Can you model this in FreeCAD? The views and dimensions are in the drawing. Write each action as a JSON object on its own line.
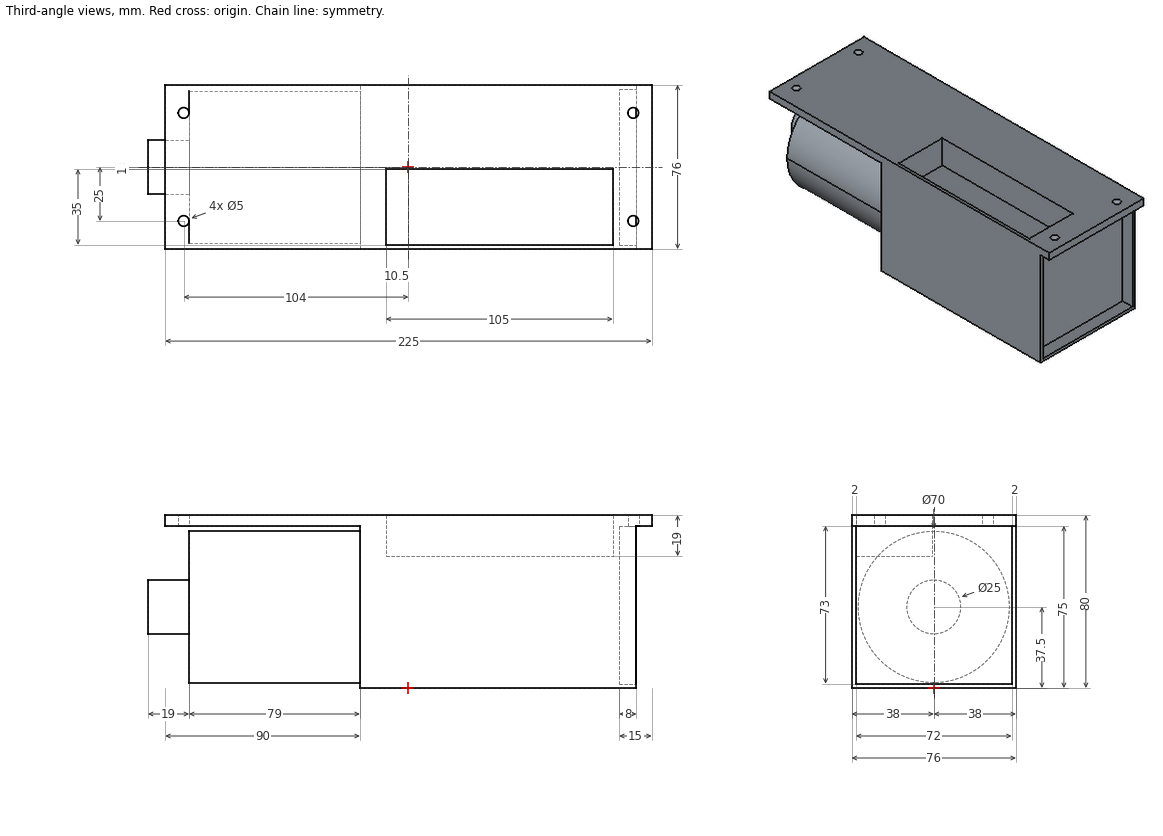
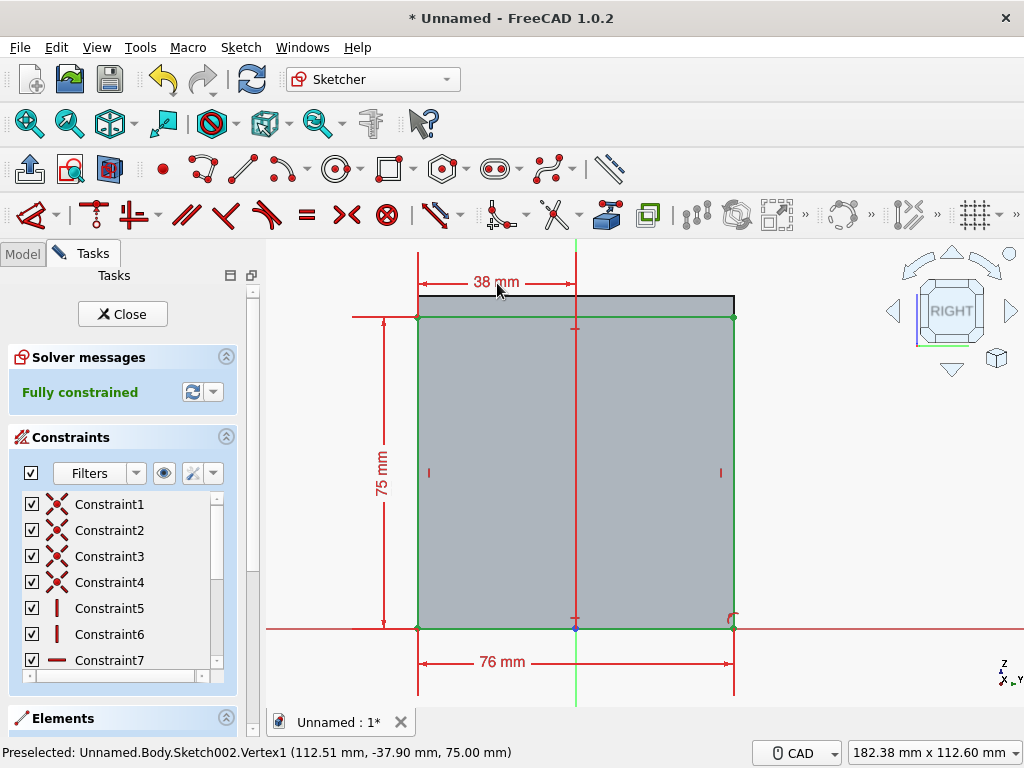
{"action": "left_click", "coordinate": [123, 314]}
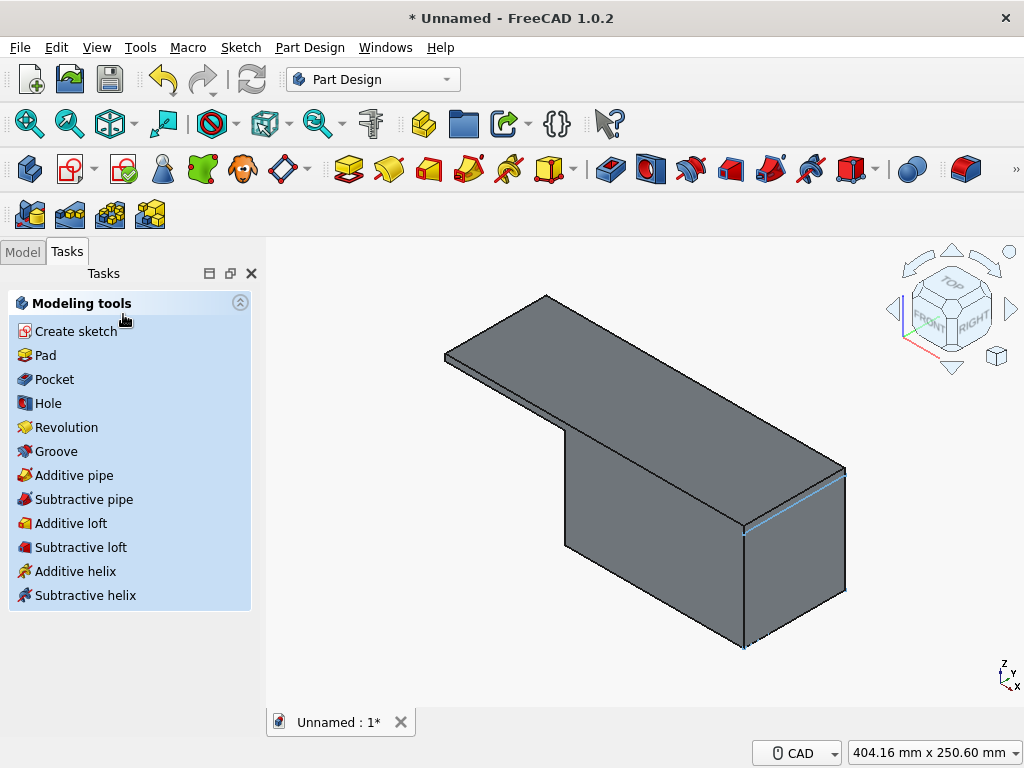
{"action": "left_click", "coordinate": [612, 170]}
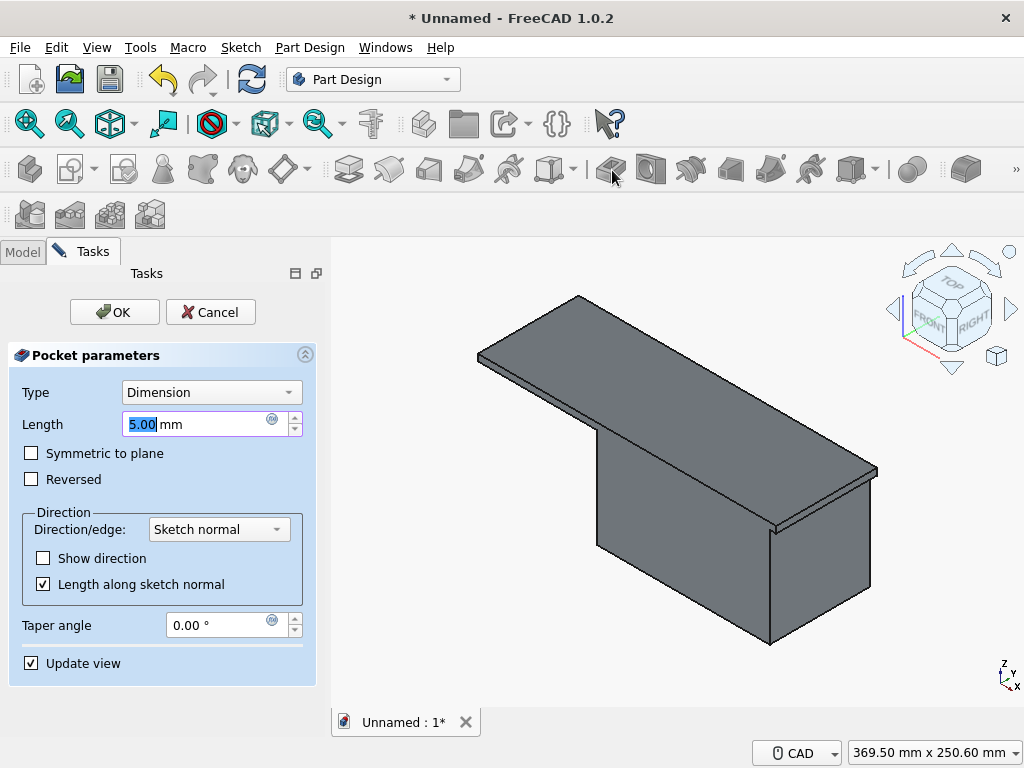
{"action": "type", "text": "15"}
{"action": "key", "text": "Tab"}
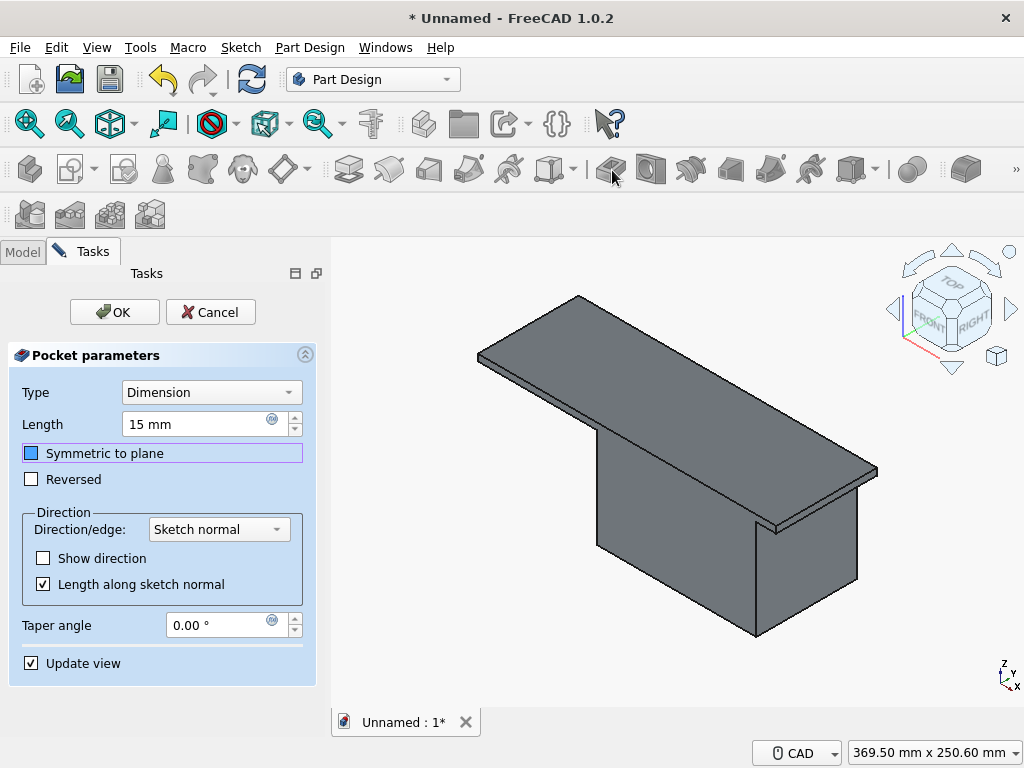
{"action": "left_click", "coordinate": [115, 312]}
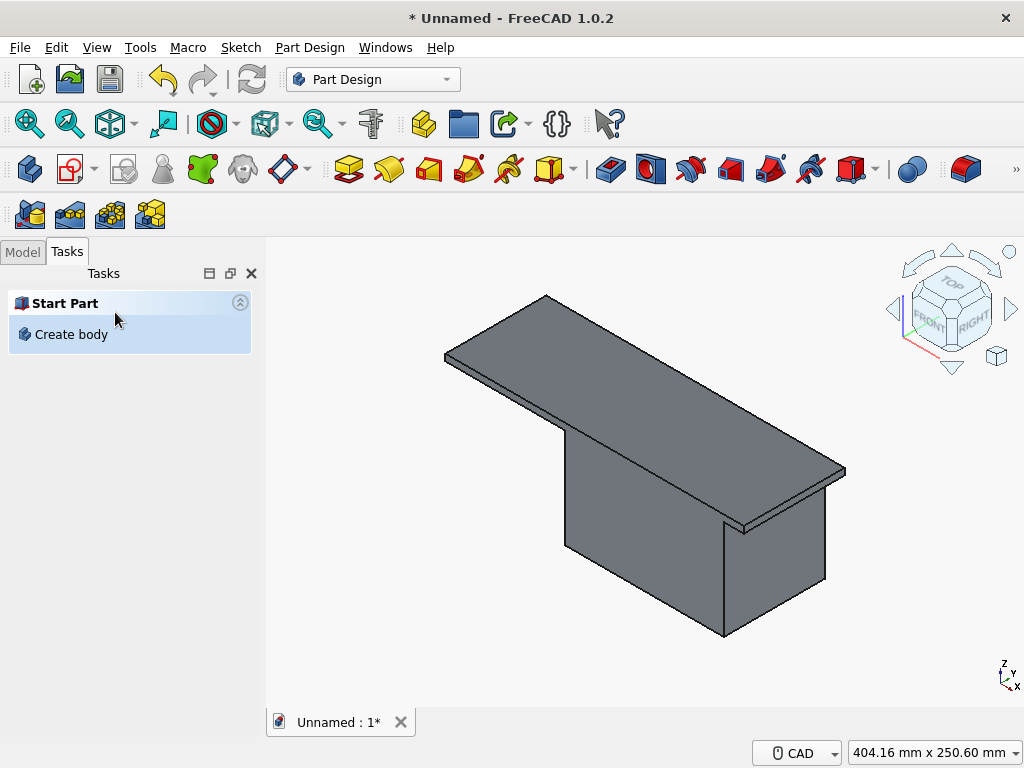
{"action": "key", "text": "5"}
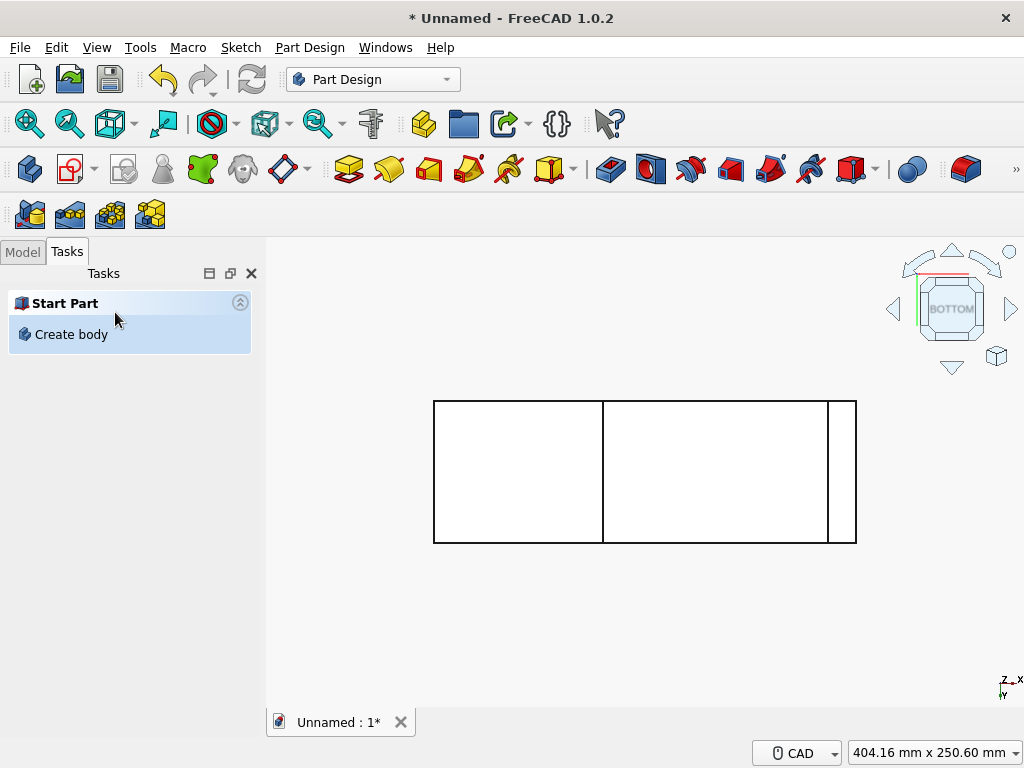
{"action": "left_click", "coordinate": [518, 471]}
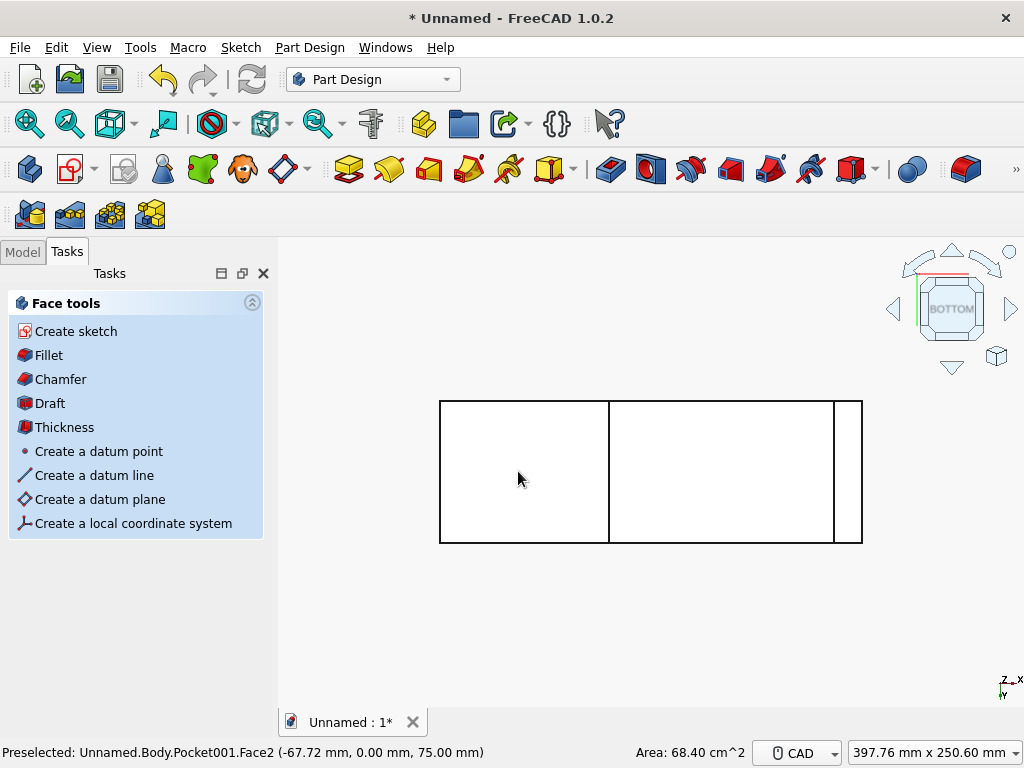
{"action": "left_click", "coordinate": [70, 170]}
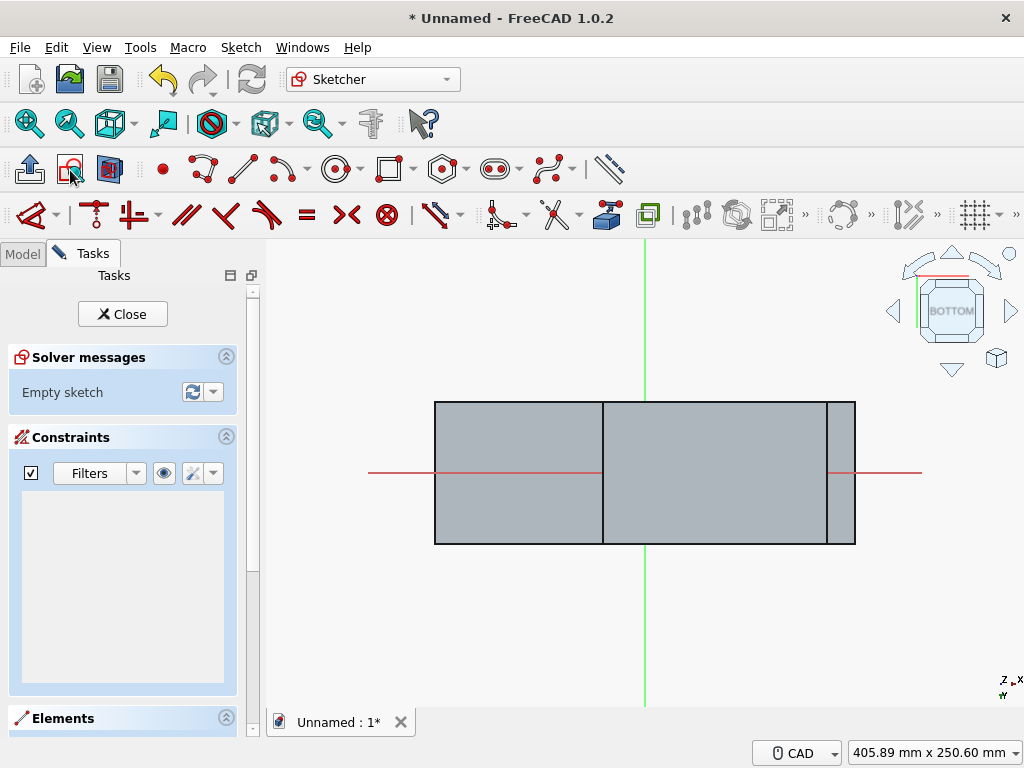
{"action": "scroll", "coordinate": [294, 473], "scroll_direction": "down", "scroll_amount": 1}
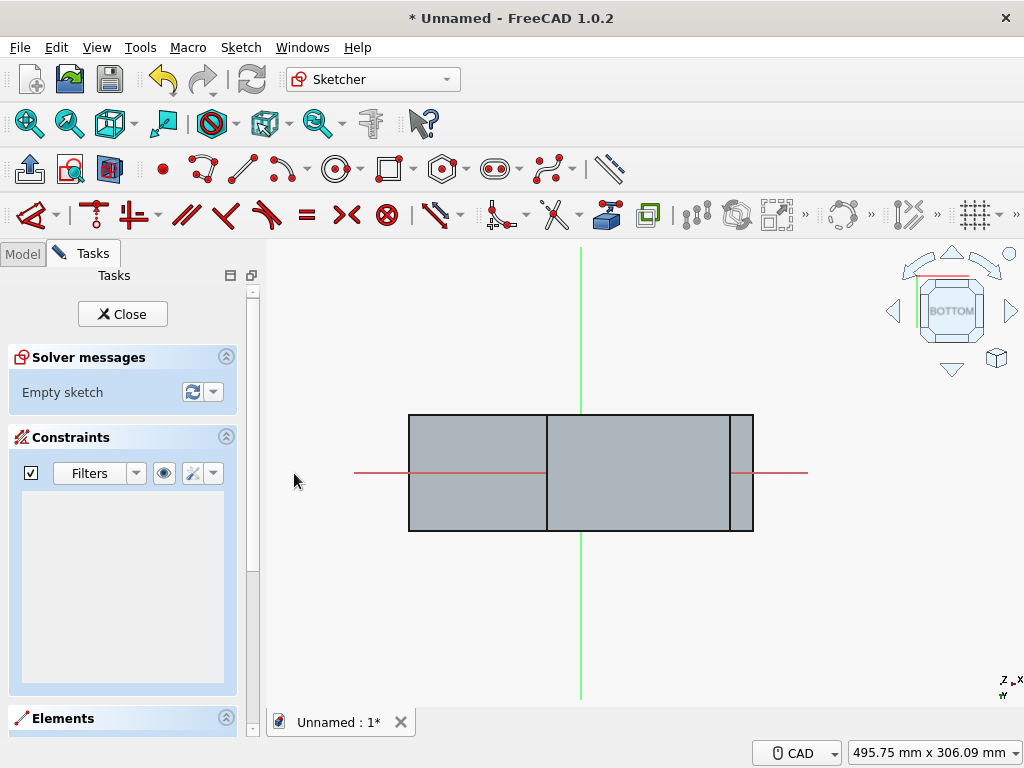
{"action": "key", "text": "g c"}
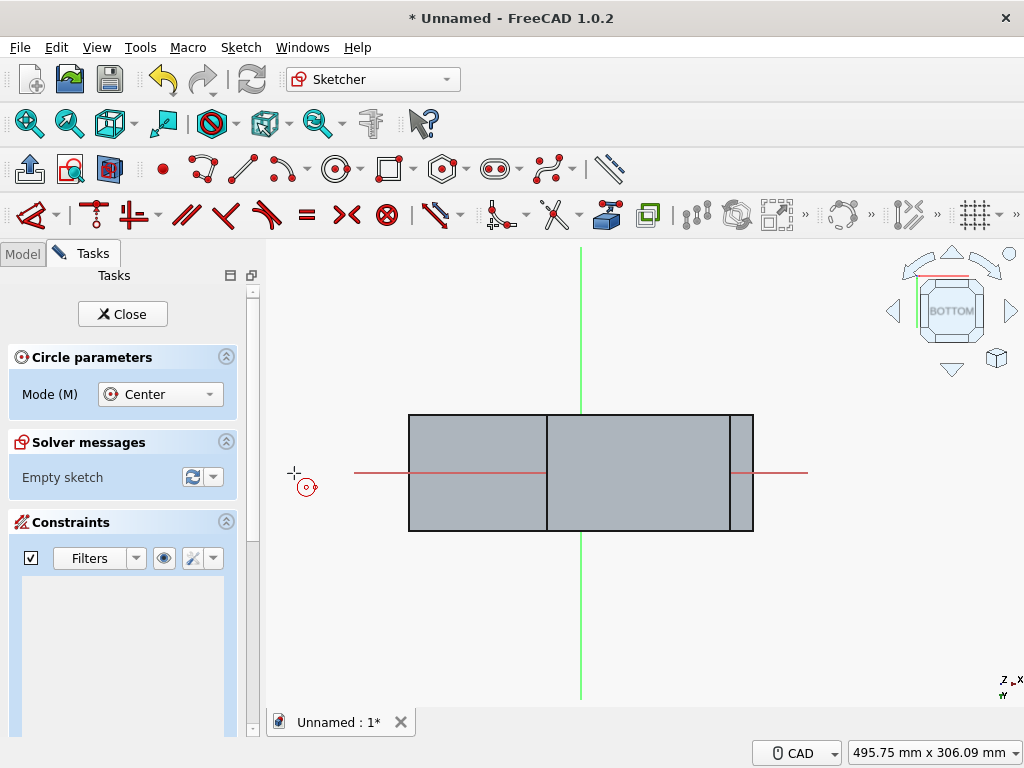
{"action": "scroll", "coordinate": [422, 435], "scroll_direction": "up", "scroll_amount": 9}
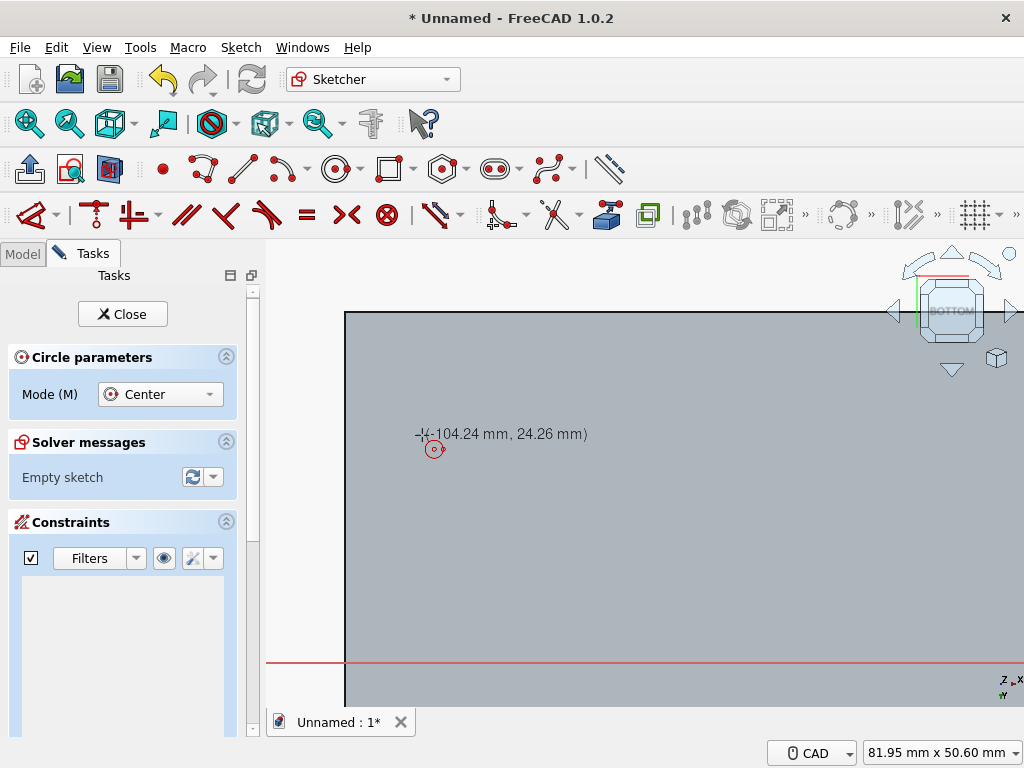
{"action": "scroll", "coordinate": [372, 425], "scroll_direction": "down", "scroll_amount": 8}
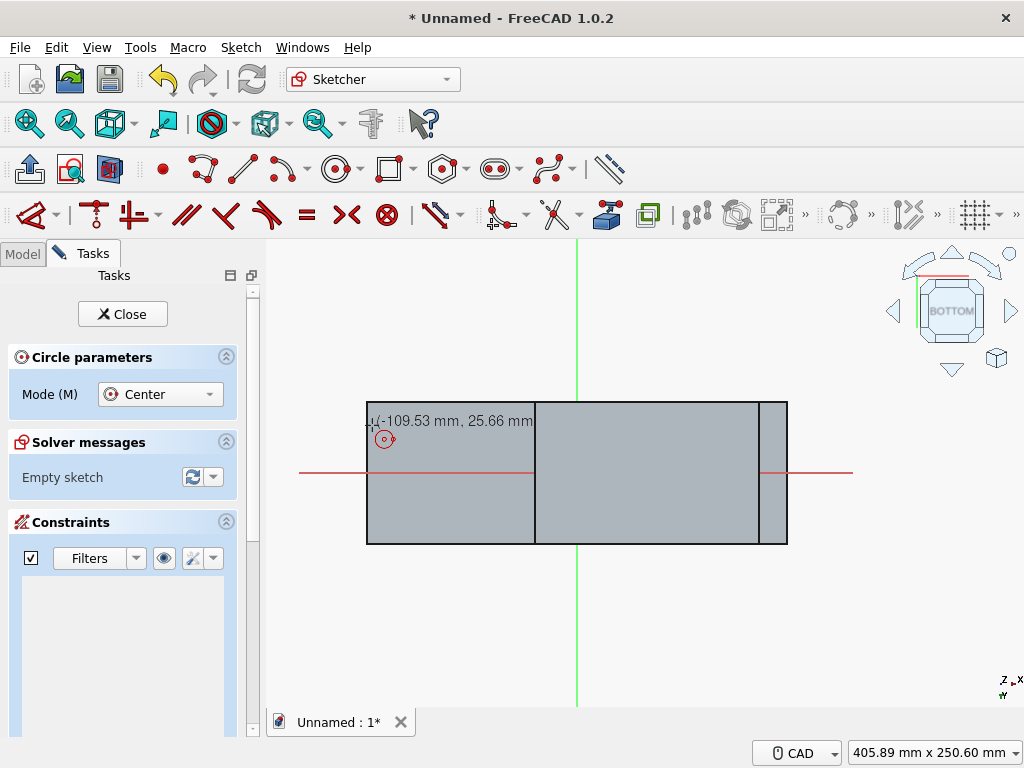
{"action": "left_click", "coordinate": [382, 427]}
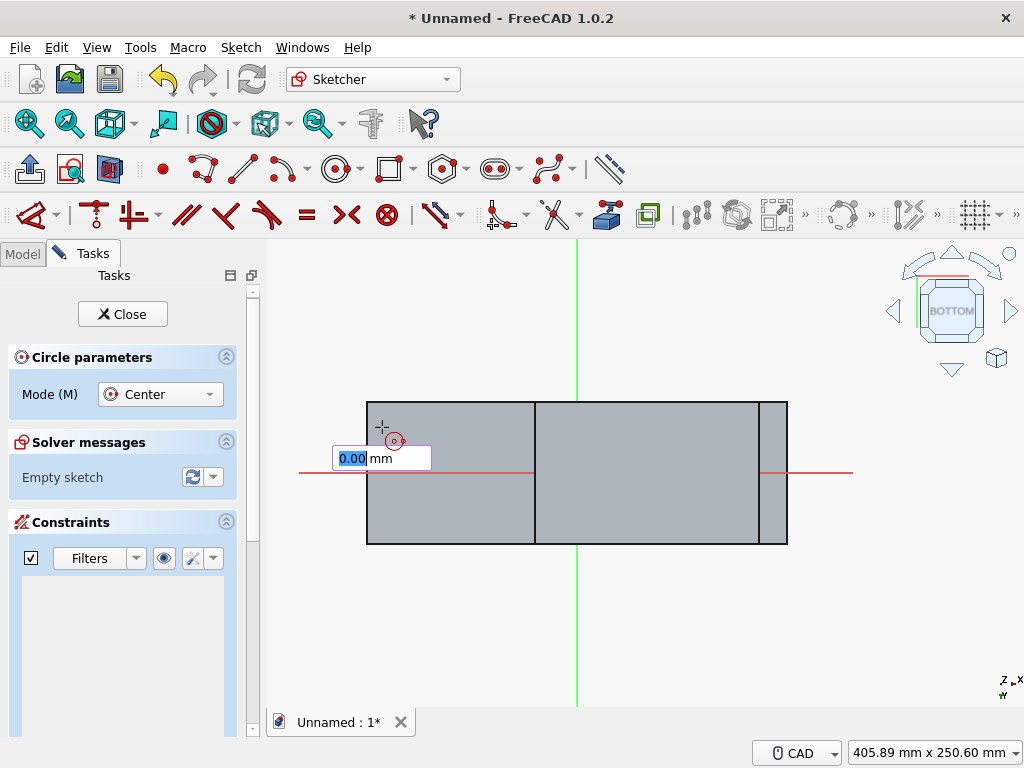
{"action": "scroll", "coordinate": [386, 423], "scroll_direction": "up", "scroll_amount": 7}